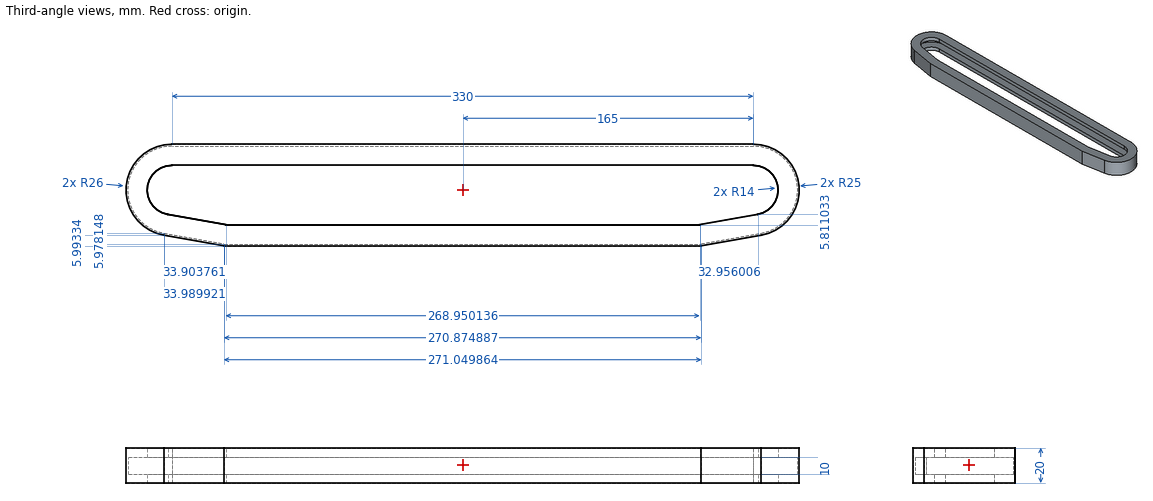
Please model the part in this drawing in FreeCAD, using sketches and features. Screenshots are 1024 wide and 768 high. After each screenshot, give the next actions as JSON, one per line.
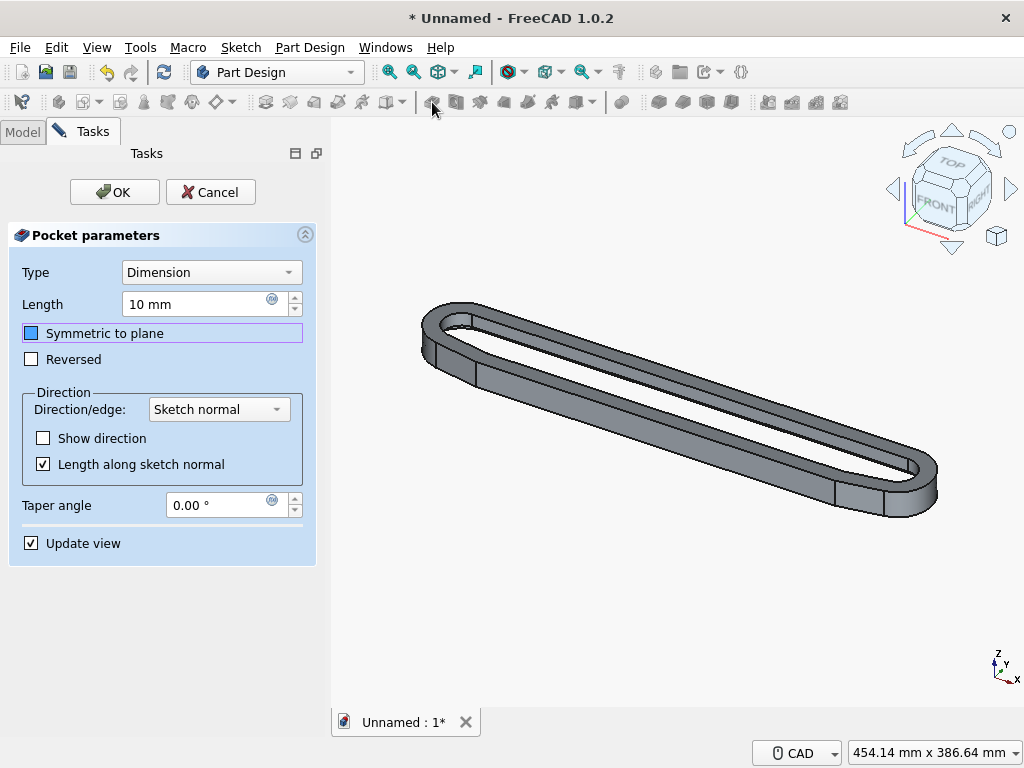
{"action": "left_click", "coordinate": [30, 333]}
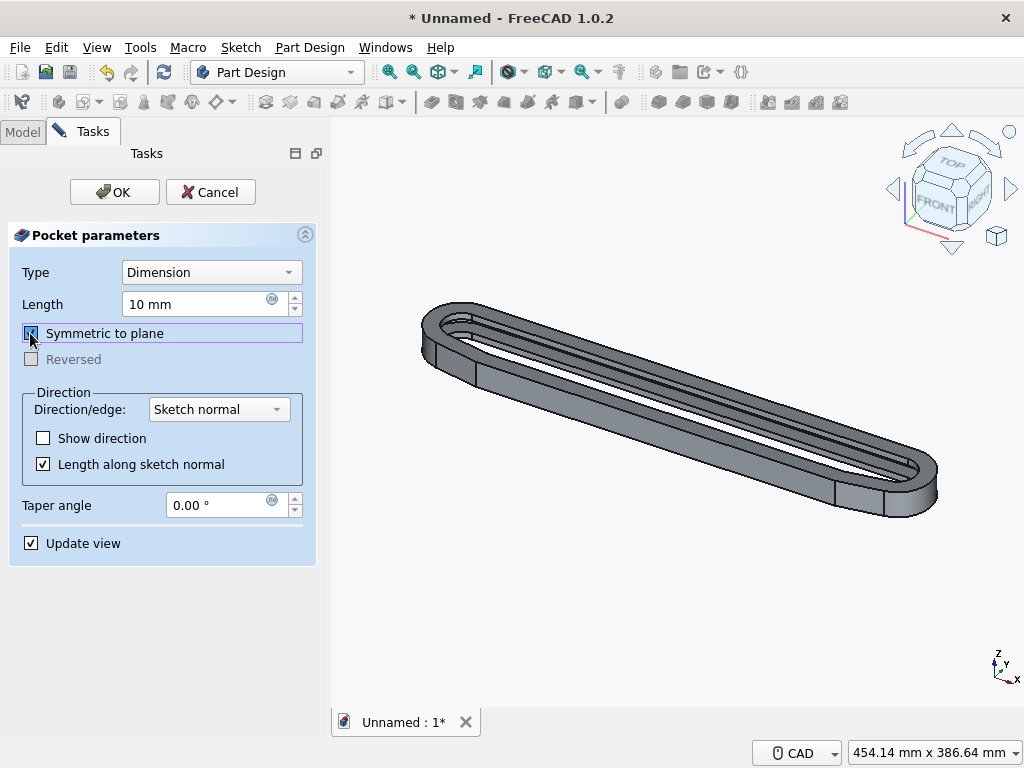
{"action": "left_click", "coordinate": [115, 192]}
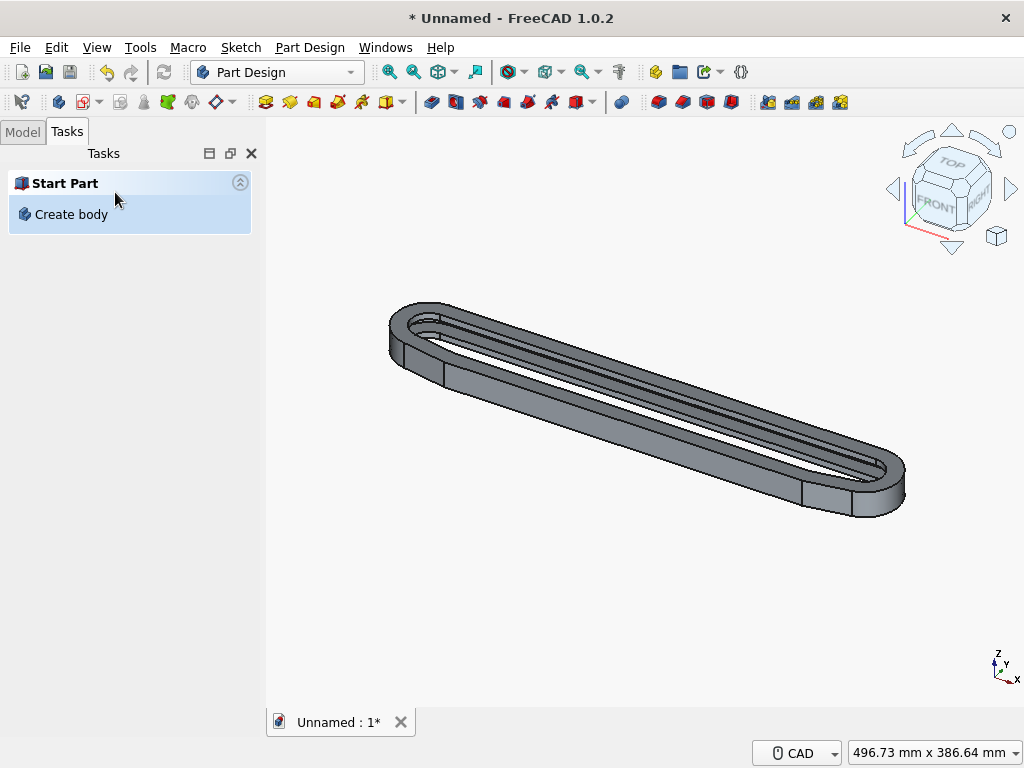
{"action": "key", "text": "0"}